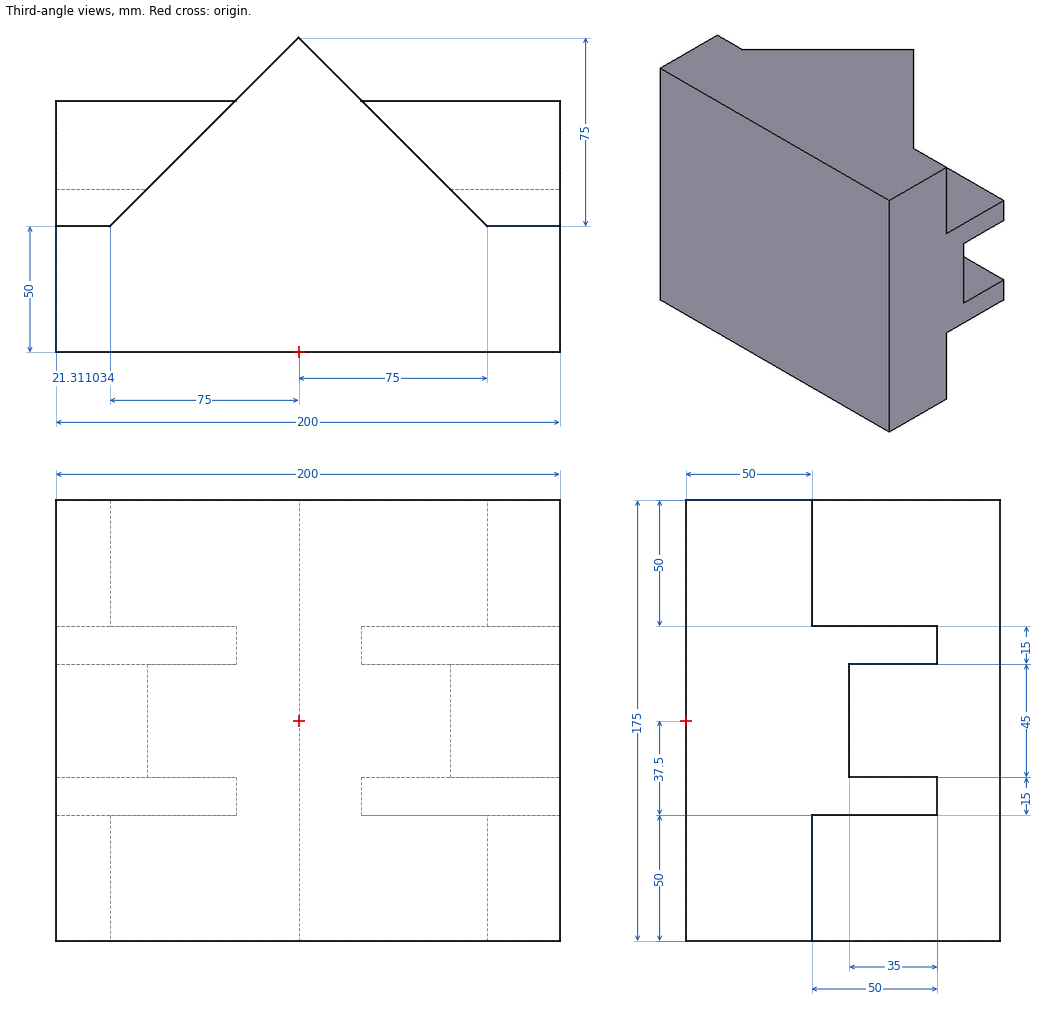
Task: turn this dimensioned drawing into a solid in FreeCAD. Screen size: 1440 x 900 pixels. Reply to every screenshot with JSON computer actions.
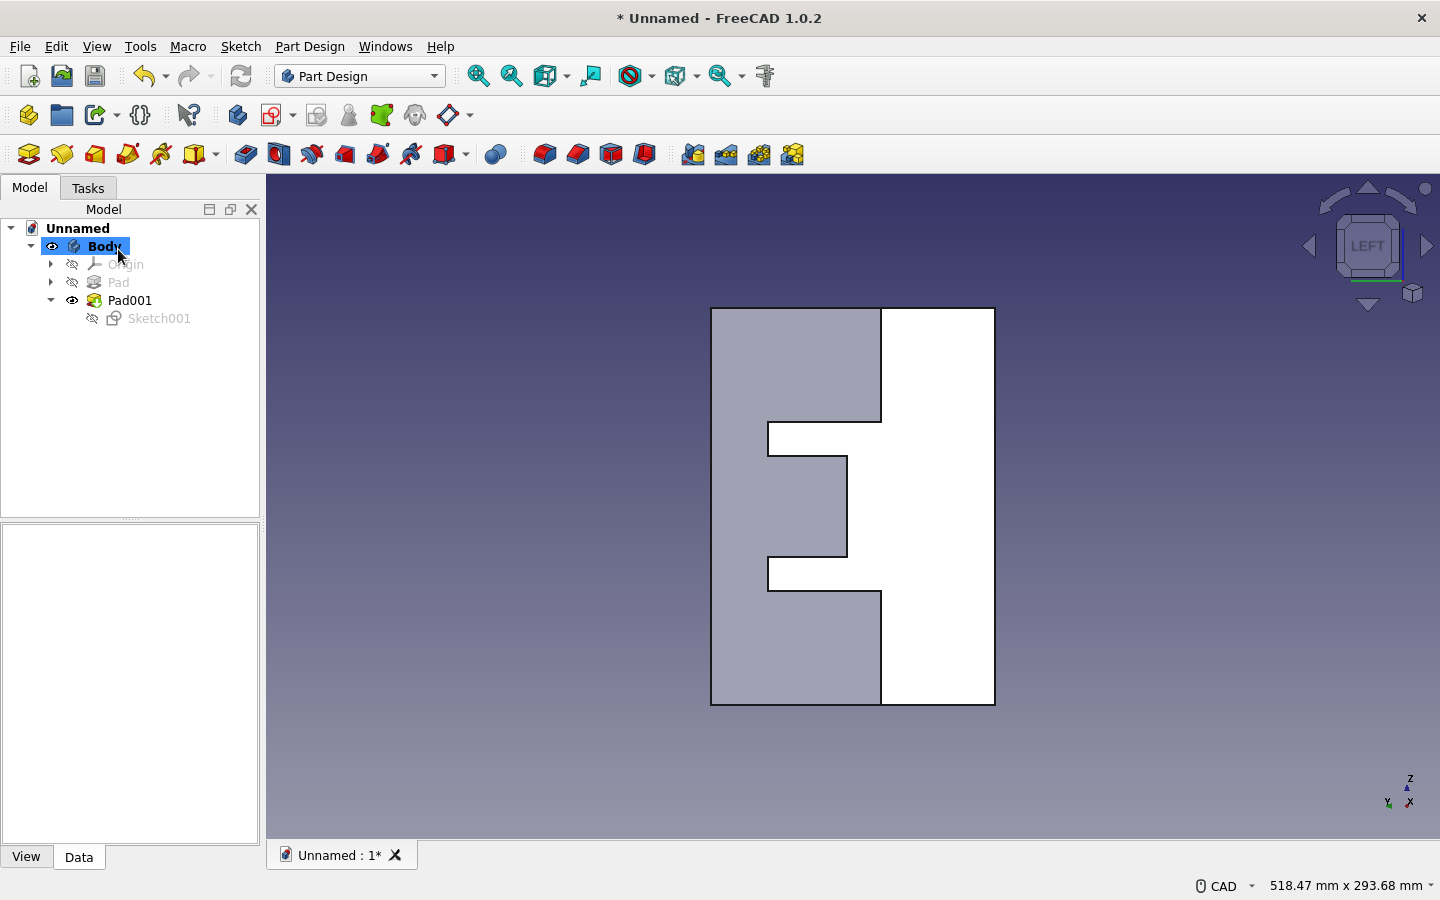
{"action": "key", "text": "0"}